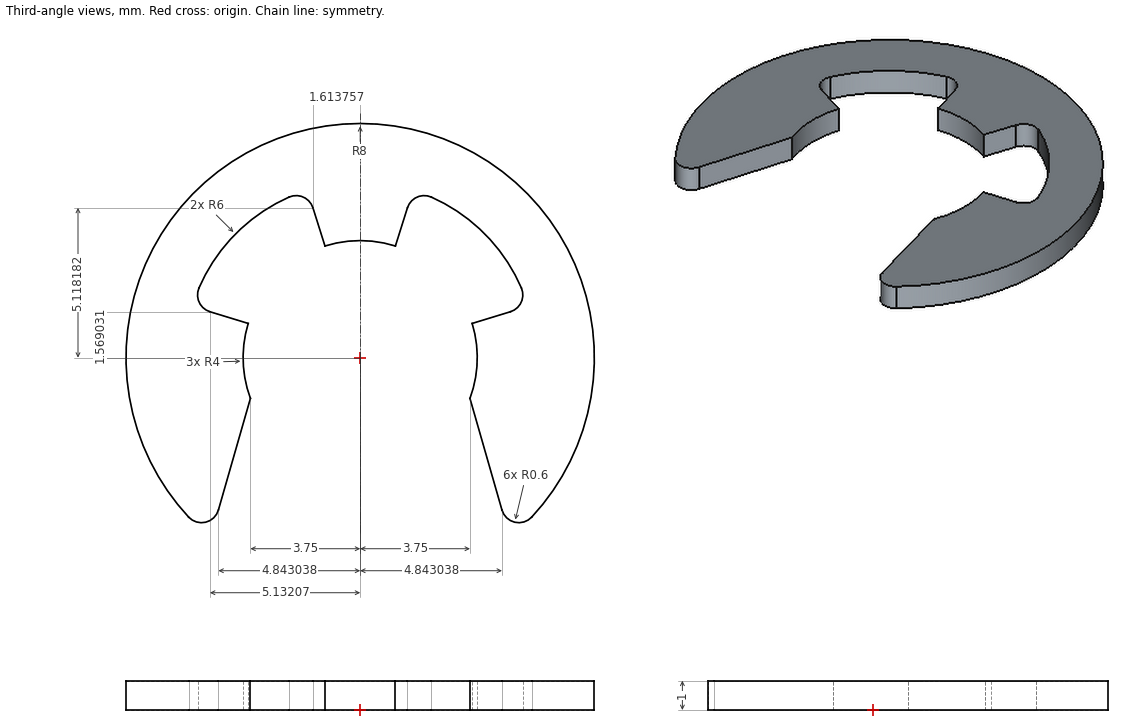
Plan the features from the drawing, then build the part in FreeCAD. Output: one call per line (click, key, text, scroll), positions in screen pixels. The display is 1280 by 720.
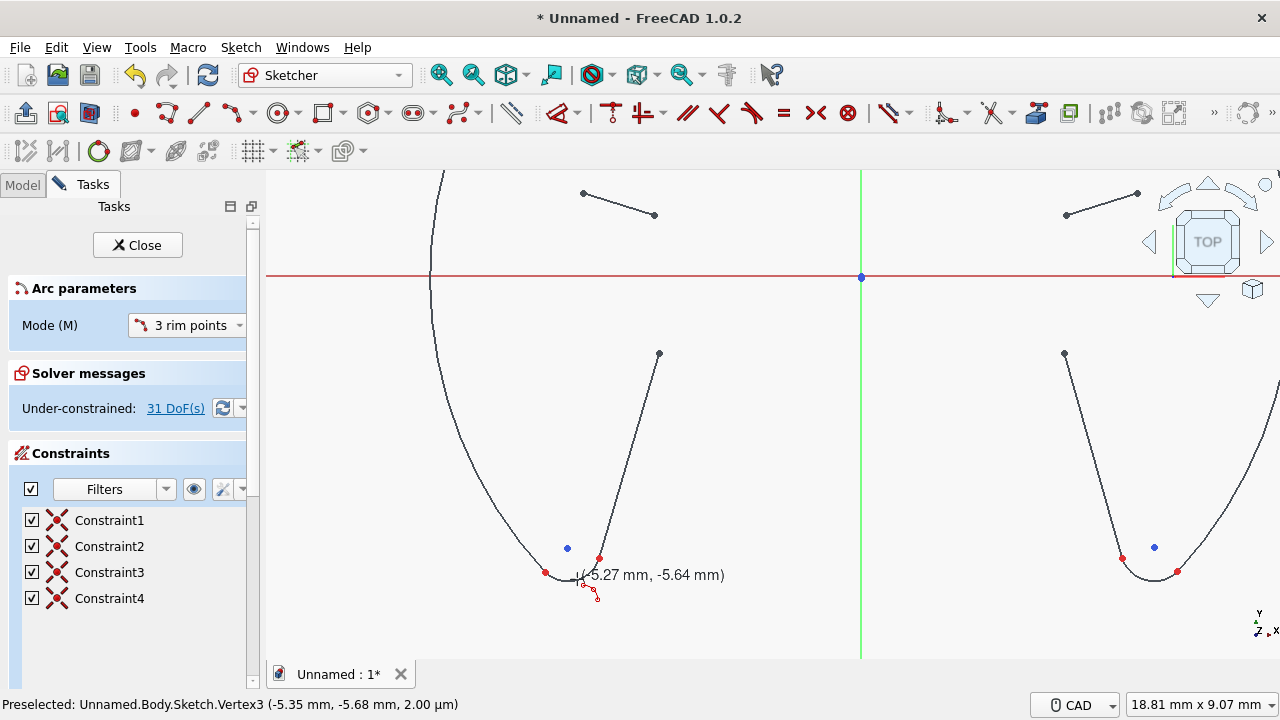
click(659, 353)
click(655, 215)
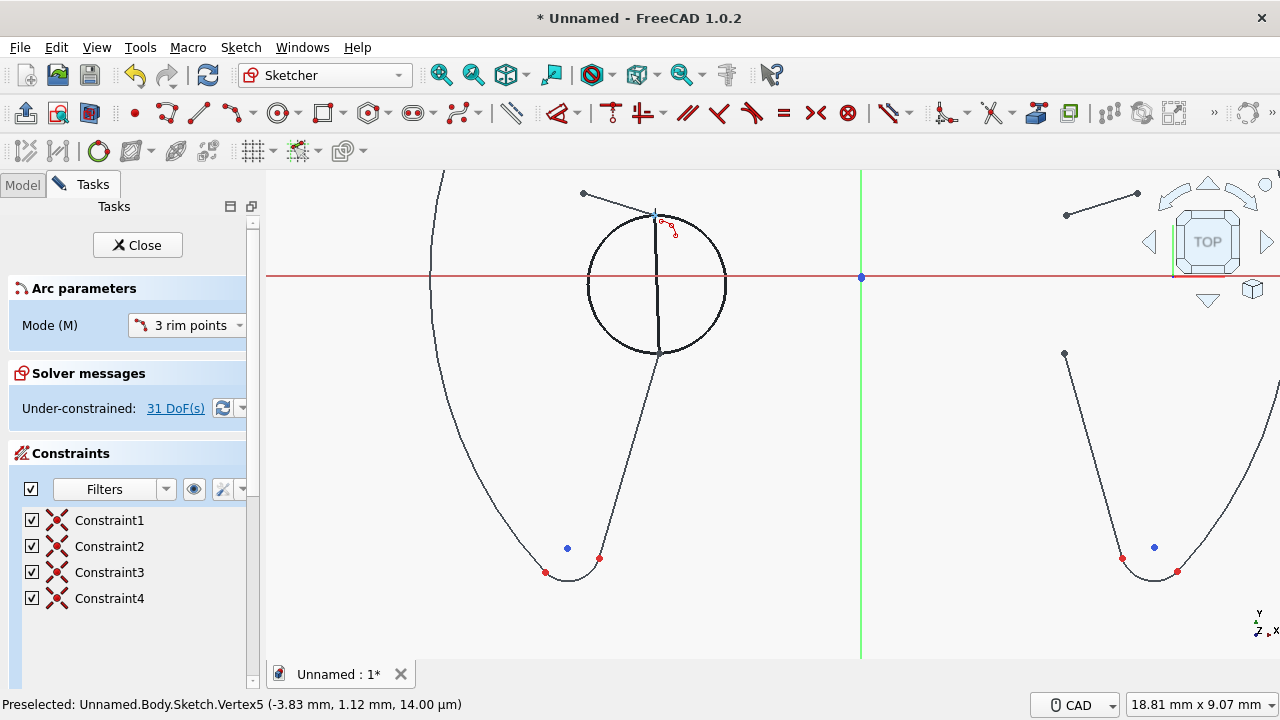
scroll(647, 296, up, 2)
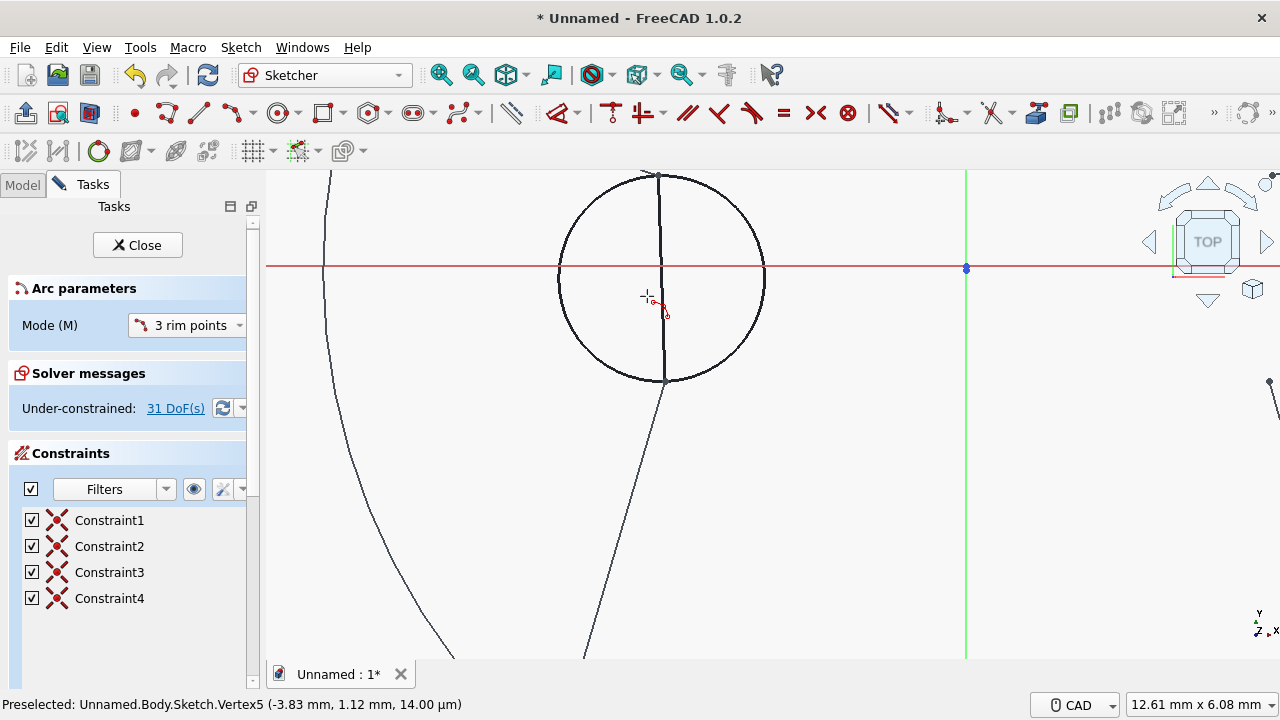
click(646, 296)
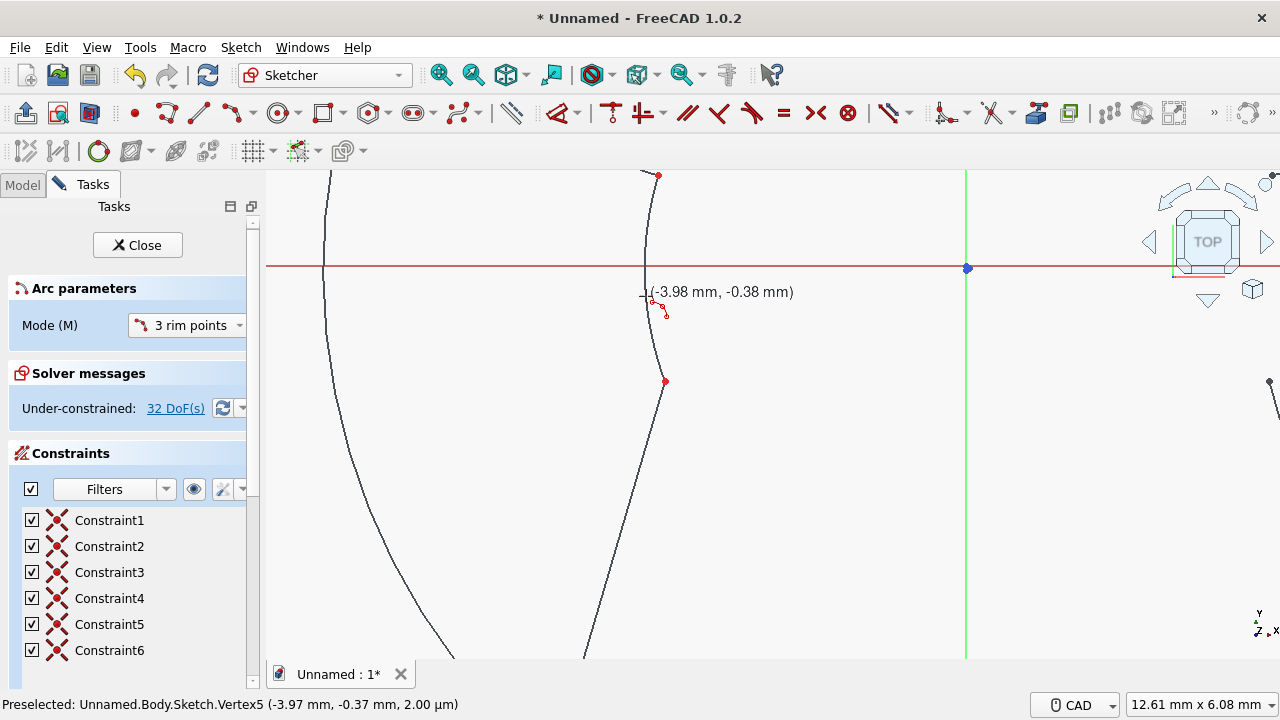
scroll(592, 520, down, 6)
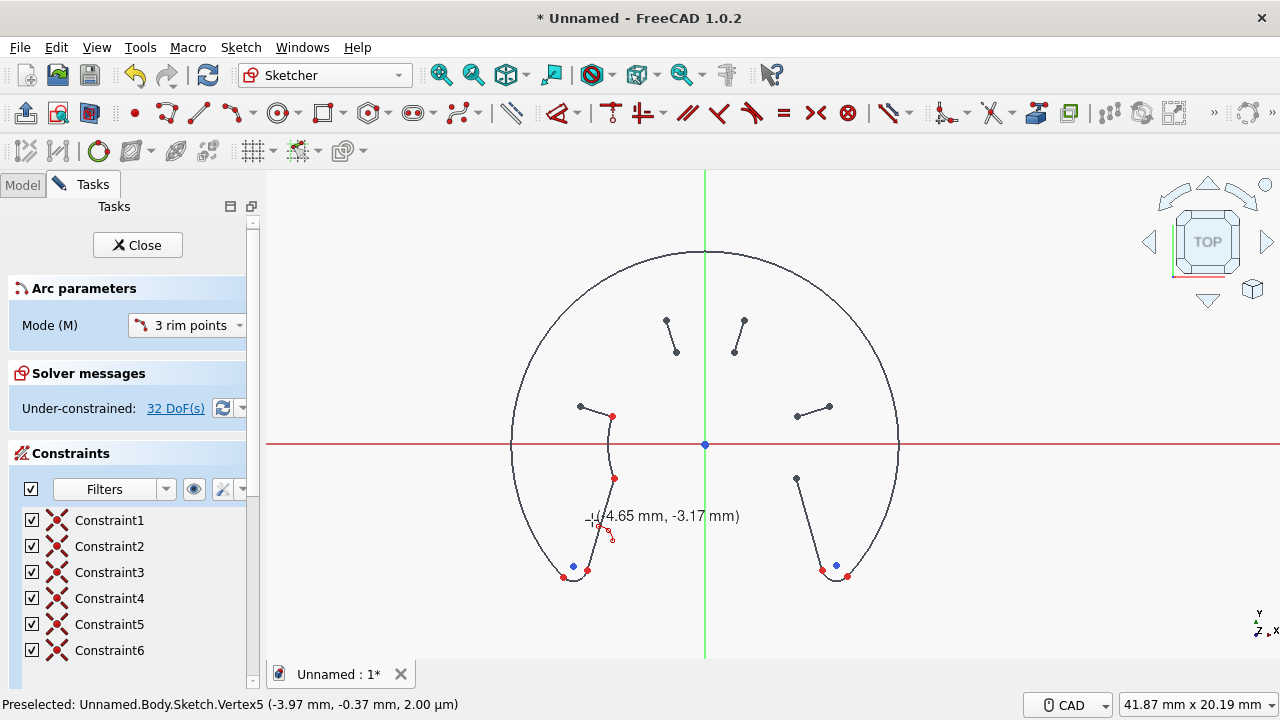
click(580, 407)
click(572, 386)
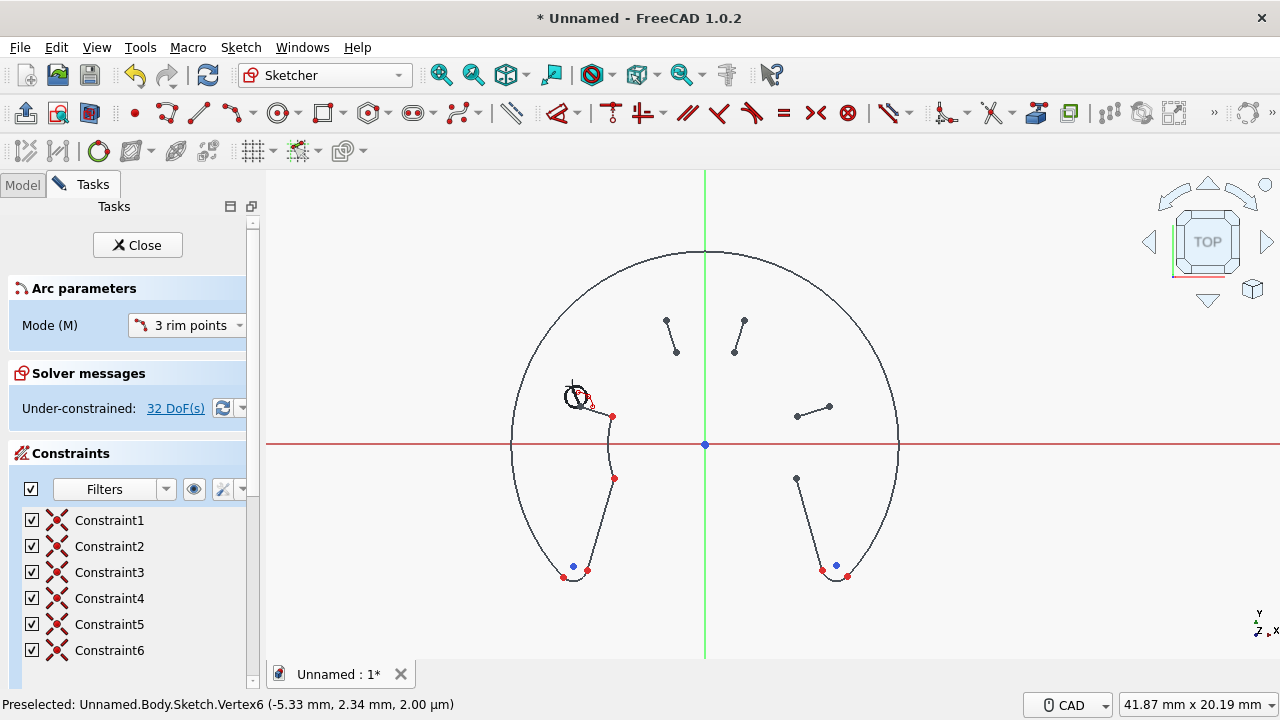
scroll(572, 398, up, 6)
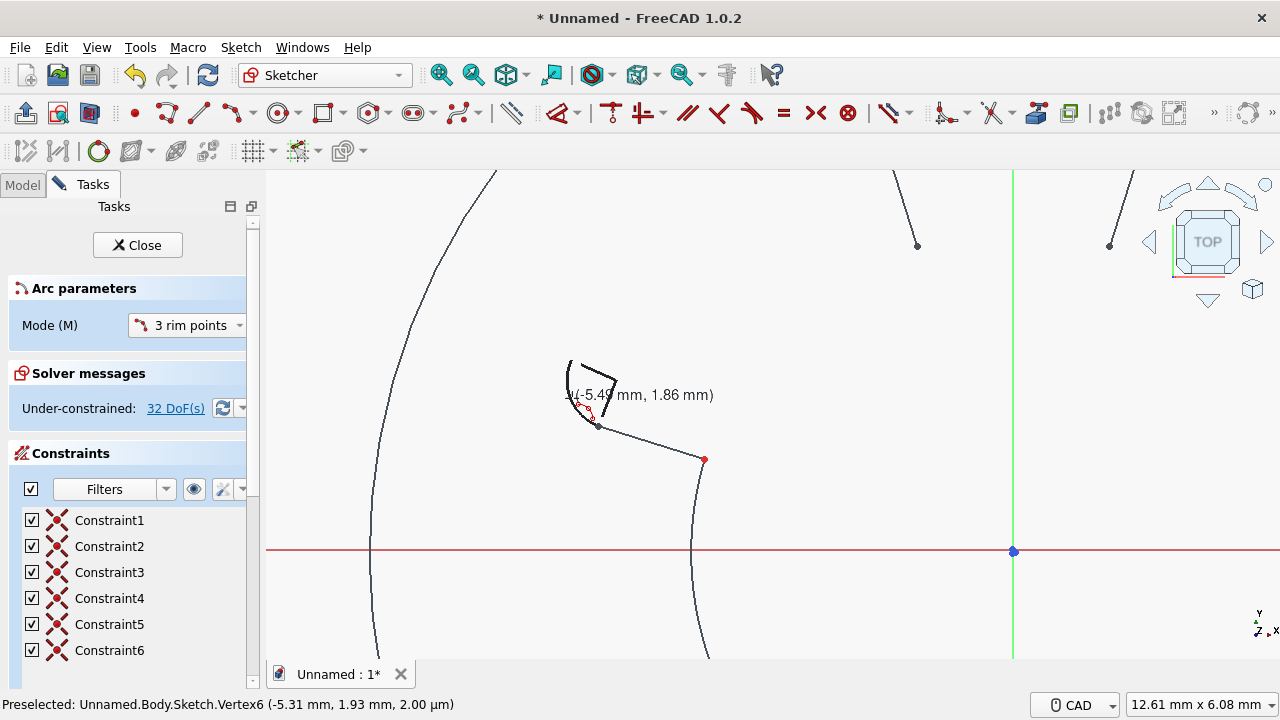
click(570, 398)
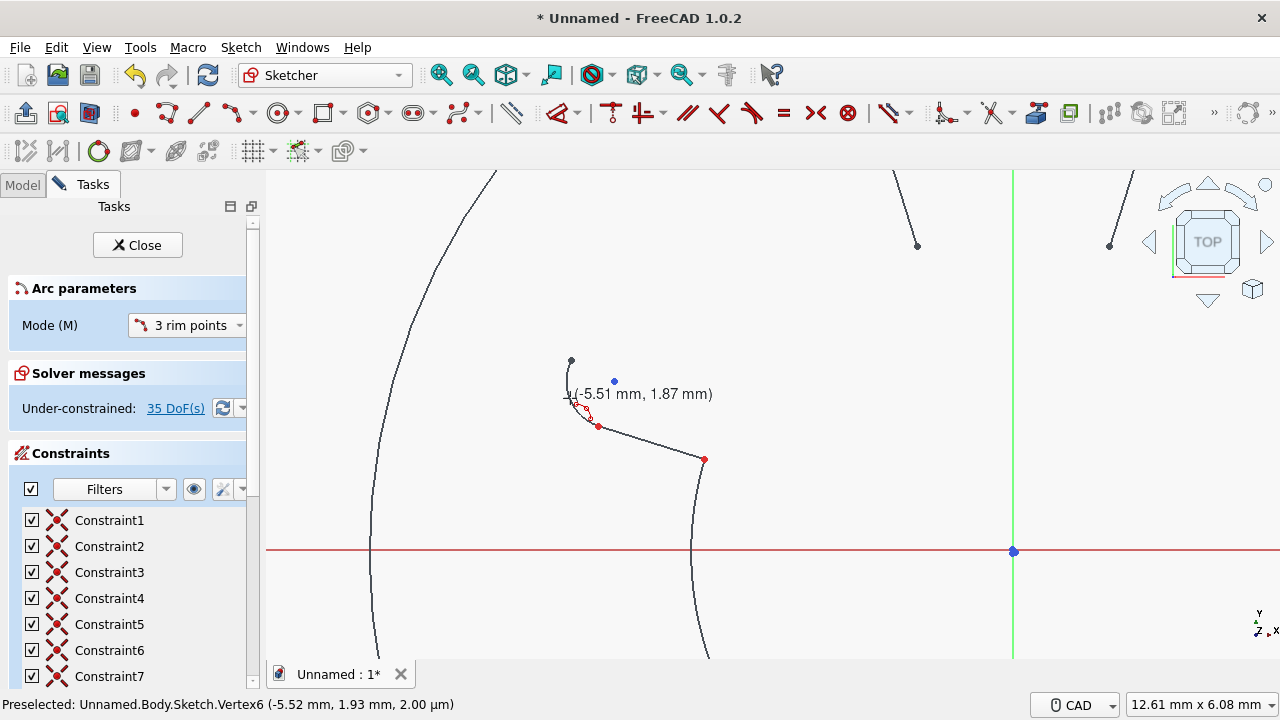
click(571, 360)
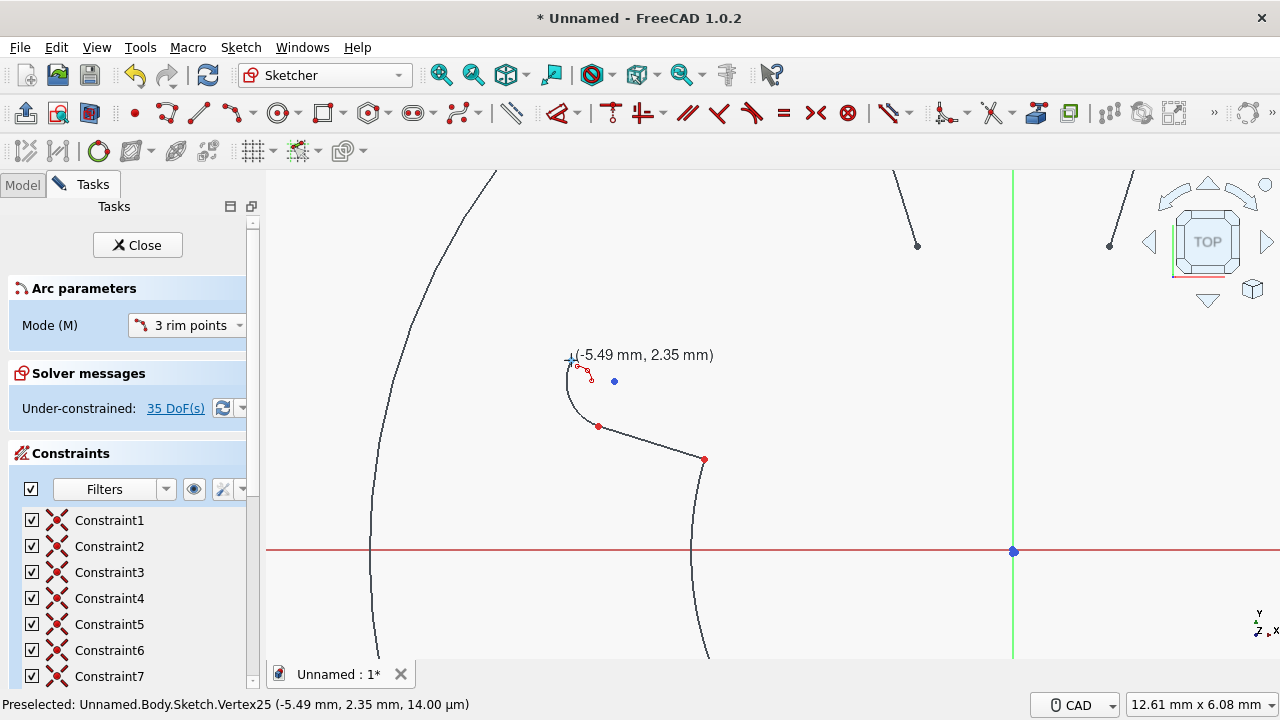
scroll(572, 397, down, 6)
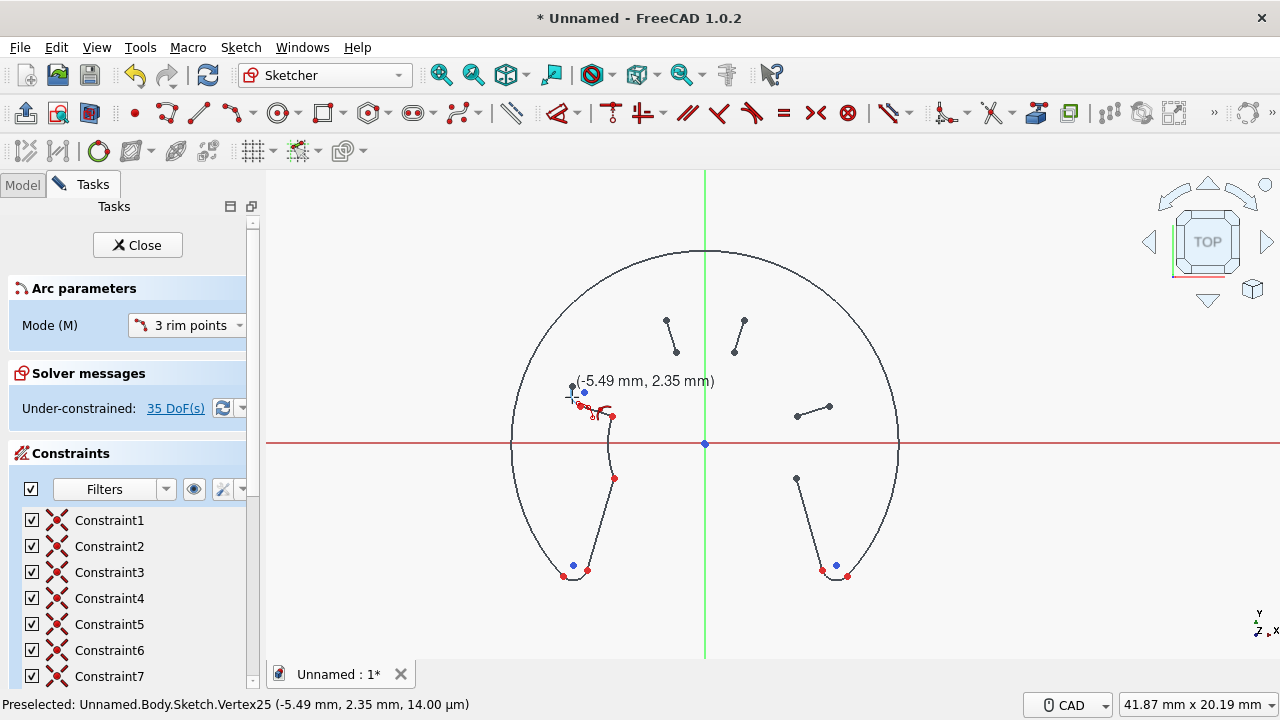
click(646, 310)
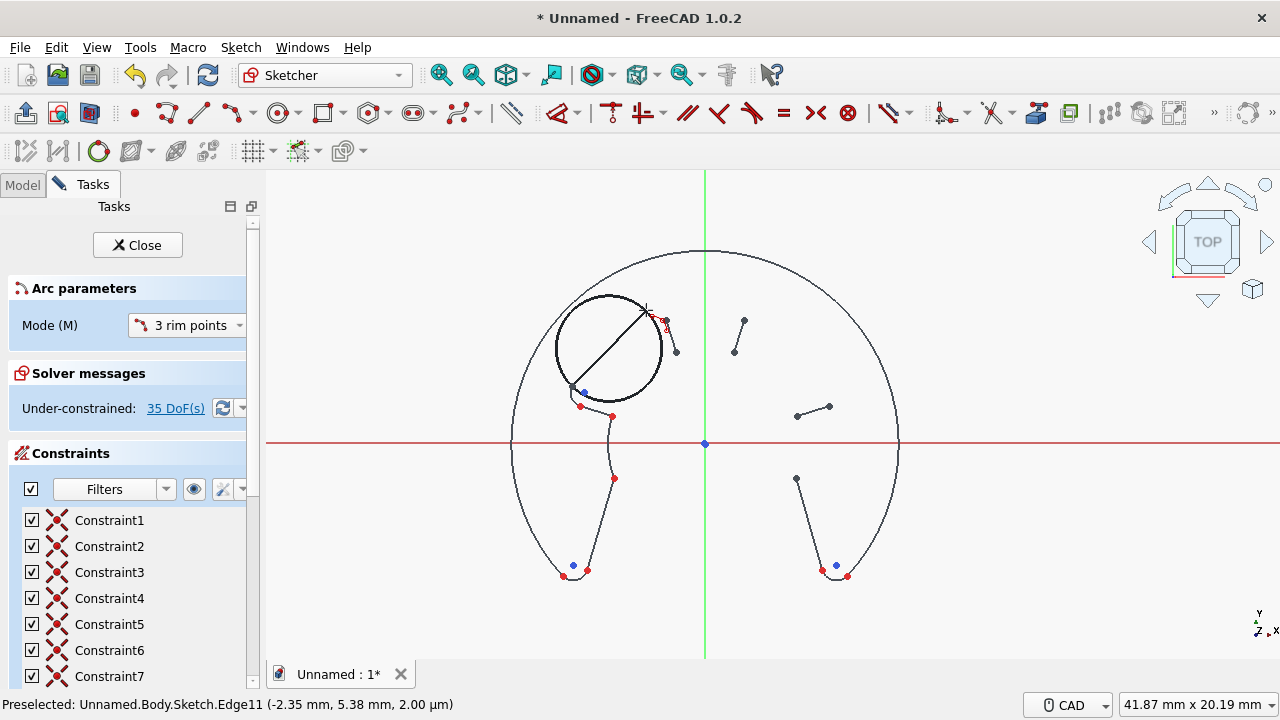
scroll(602, 341, up, 3)